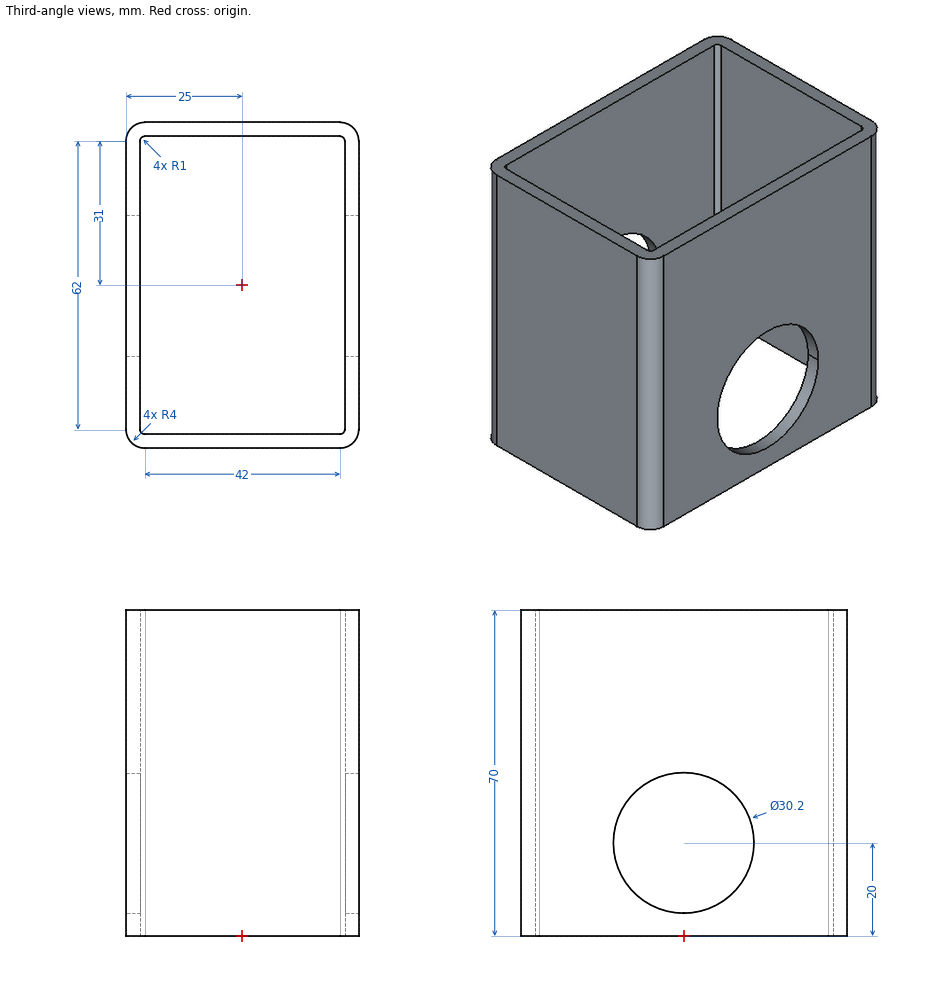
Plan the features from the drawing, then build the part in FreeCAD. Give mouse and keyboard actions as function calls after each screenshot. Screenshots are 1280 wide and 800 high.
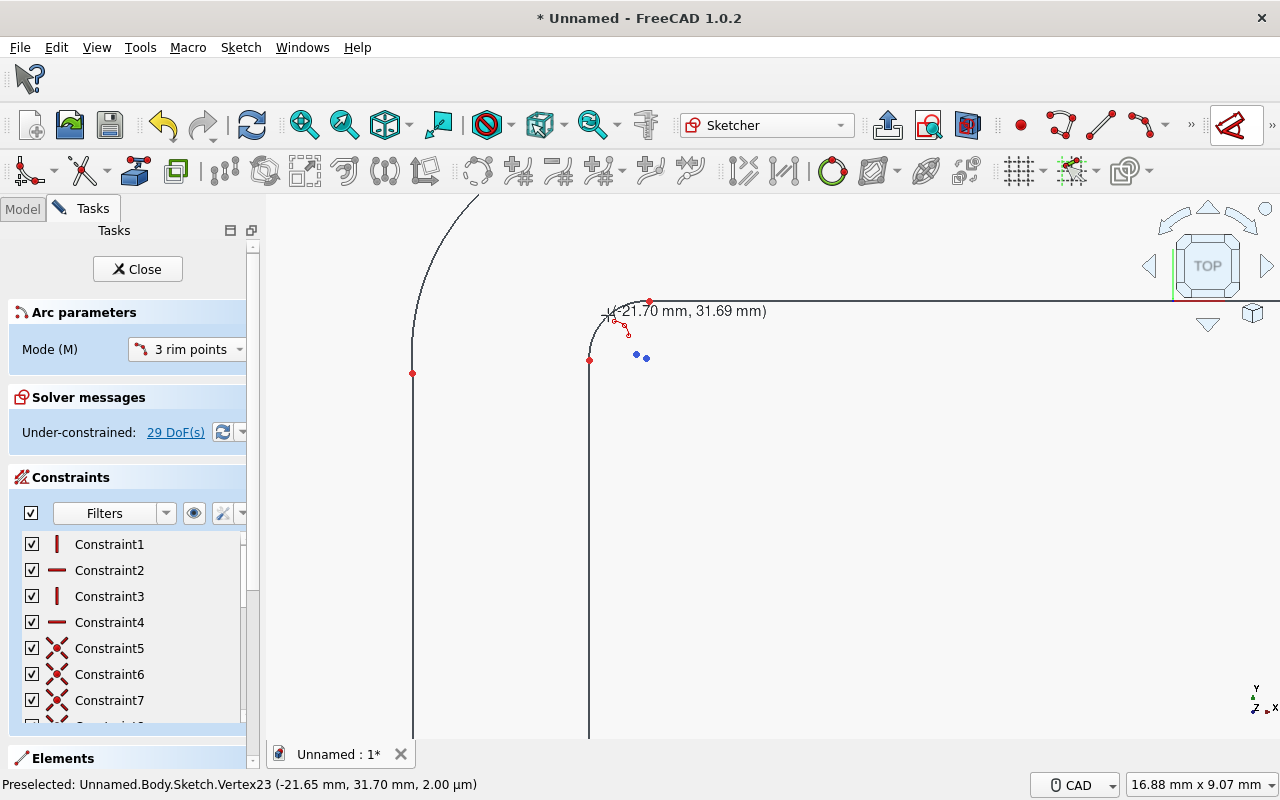
scroll(608, 326, down, 13)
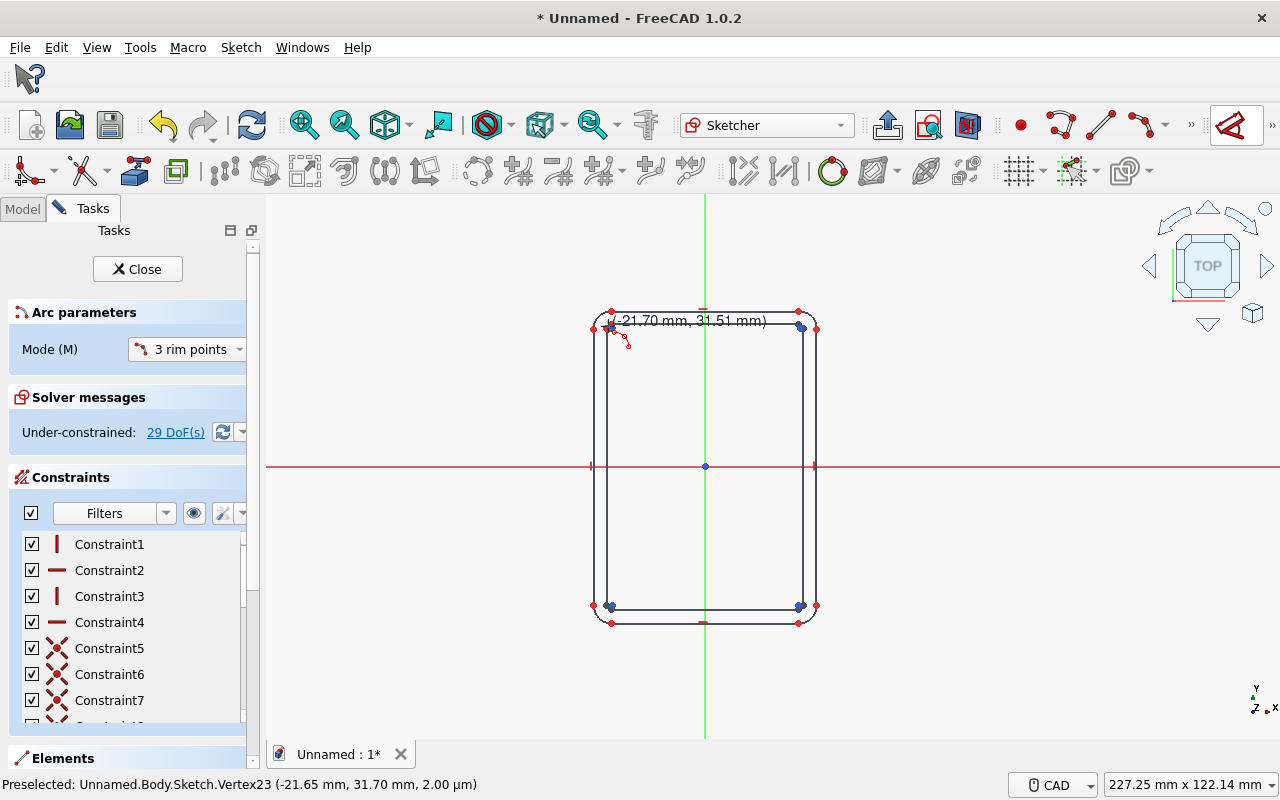
scroll(799, 324, up, 7)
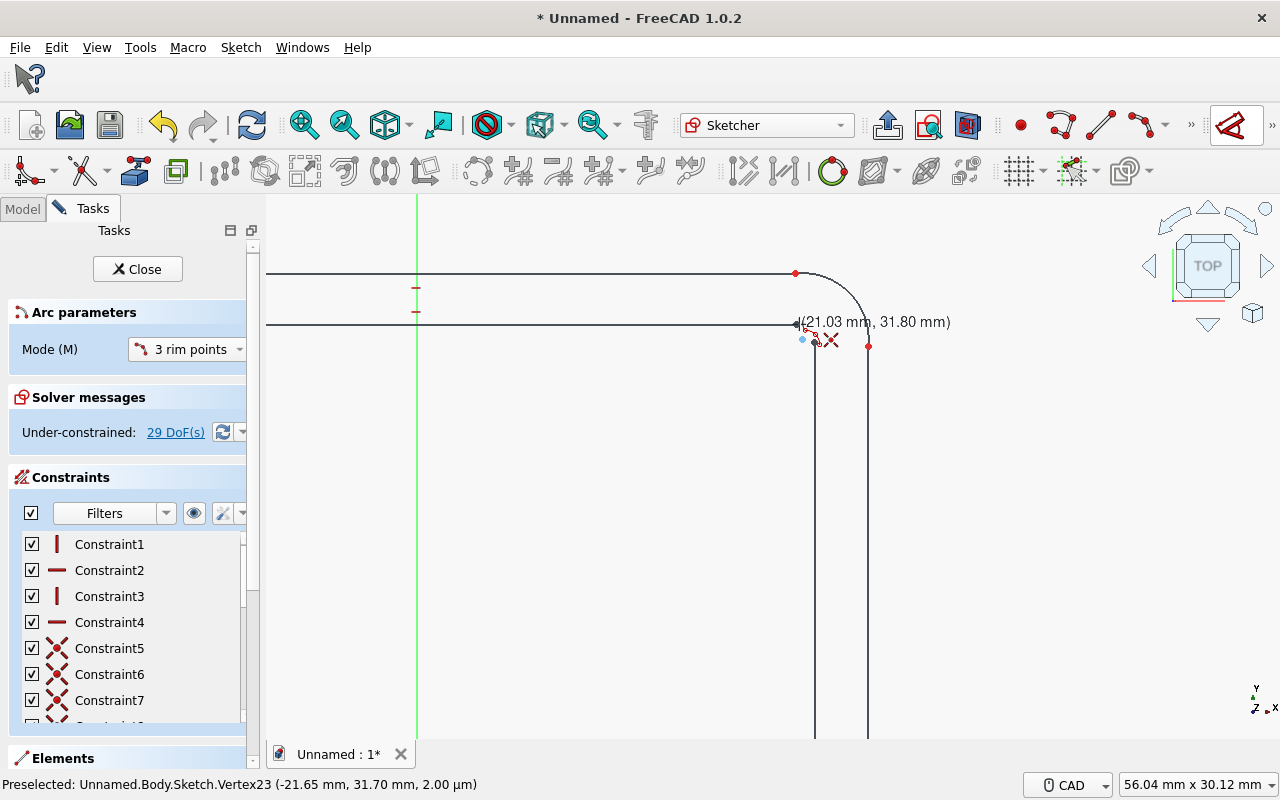
click(797, 325)
click(815, 343)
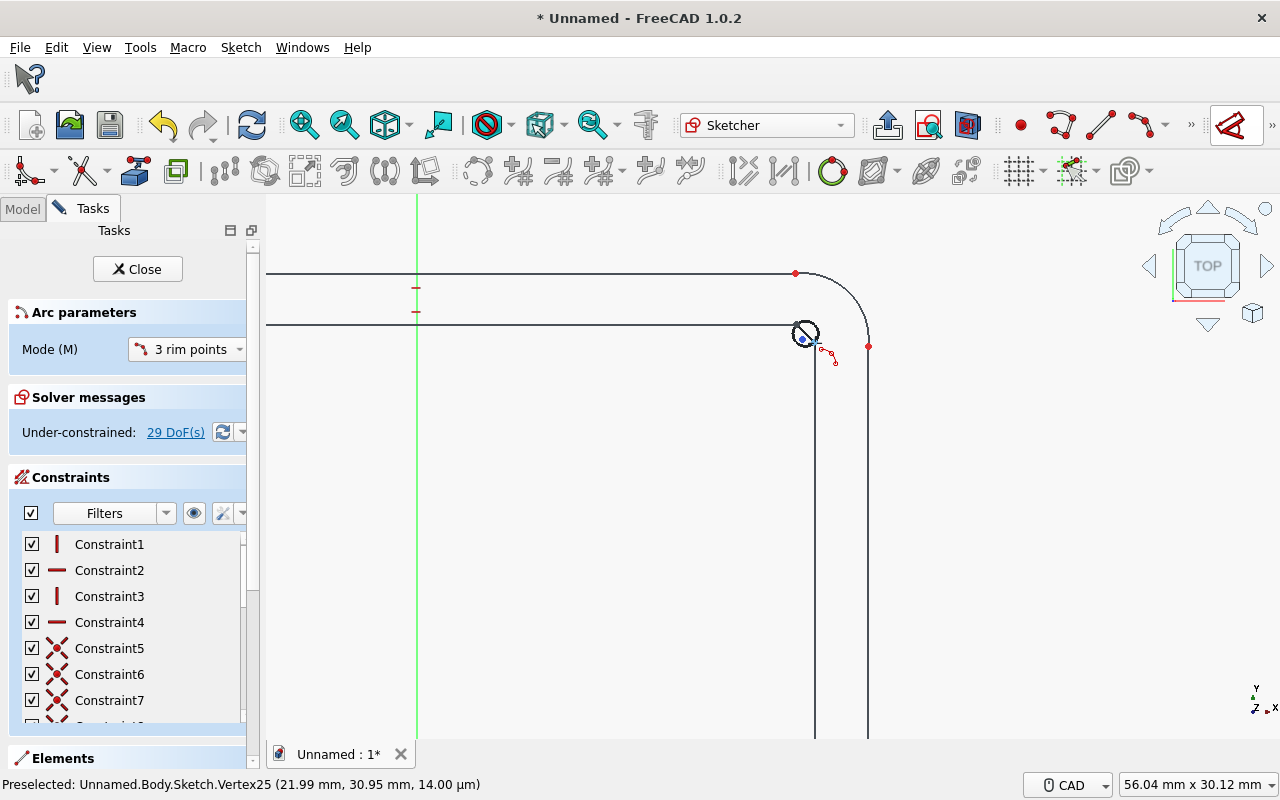
scroll(810, 329, up, 6)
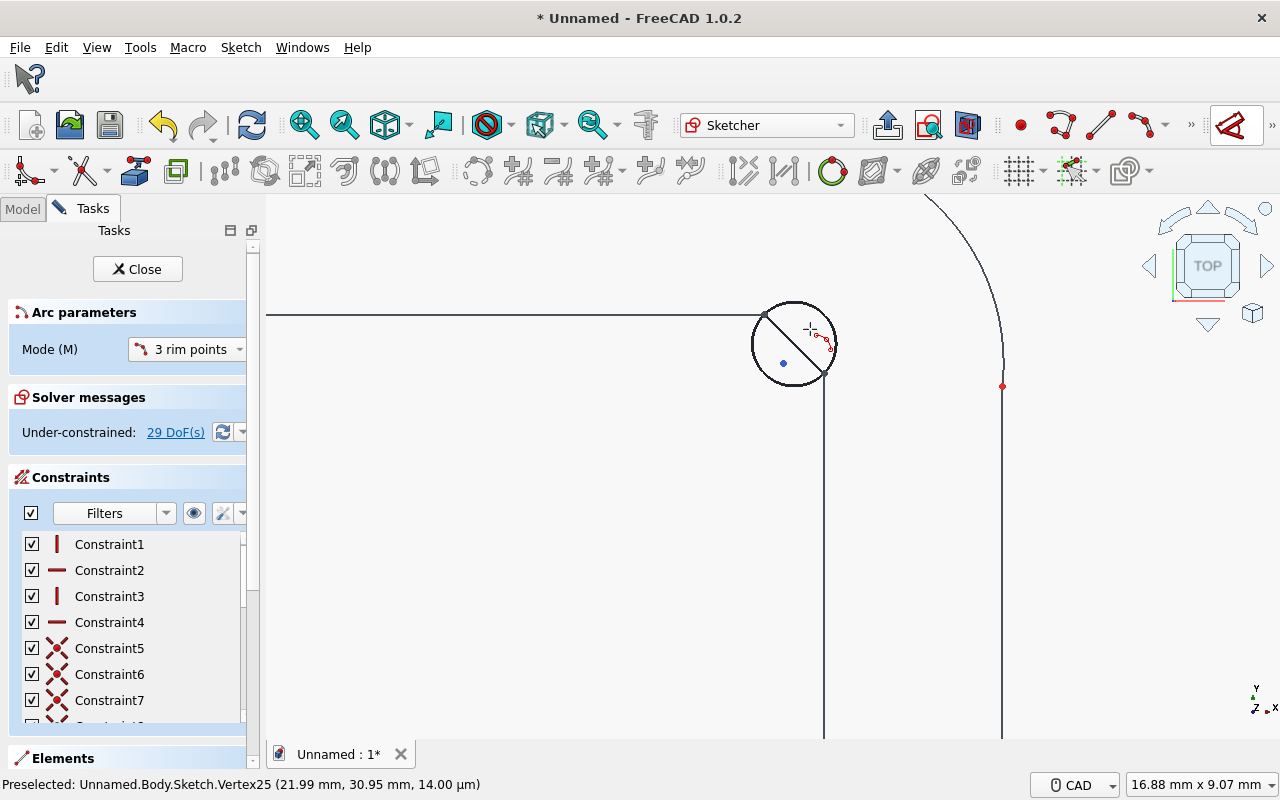
click(807, 328)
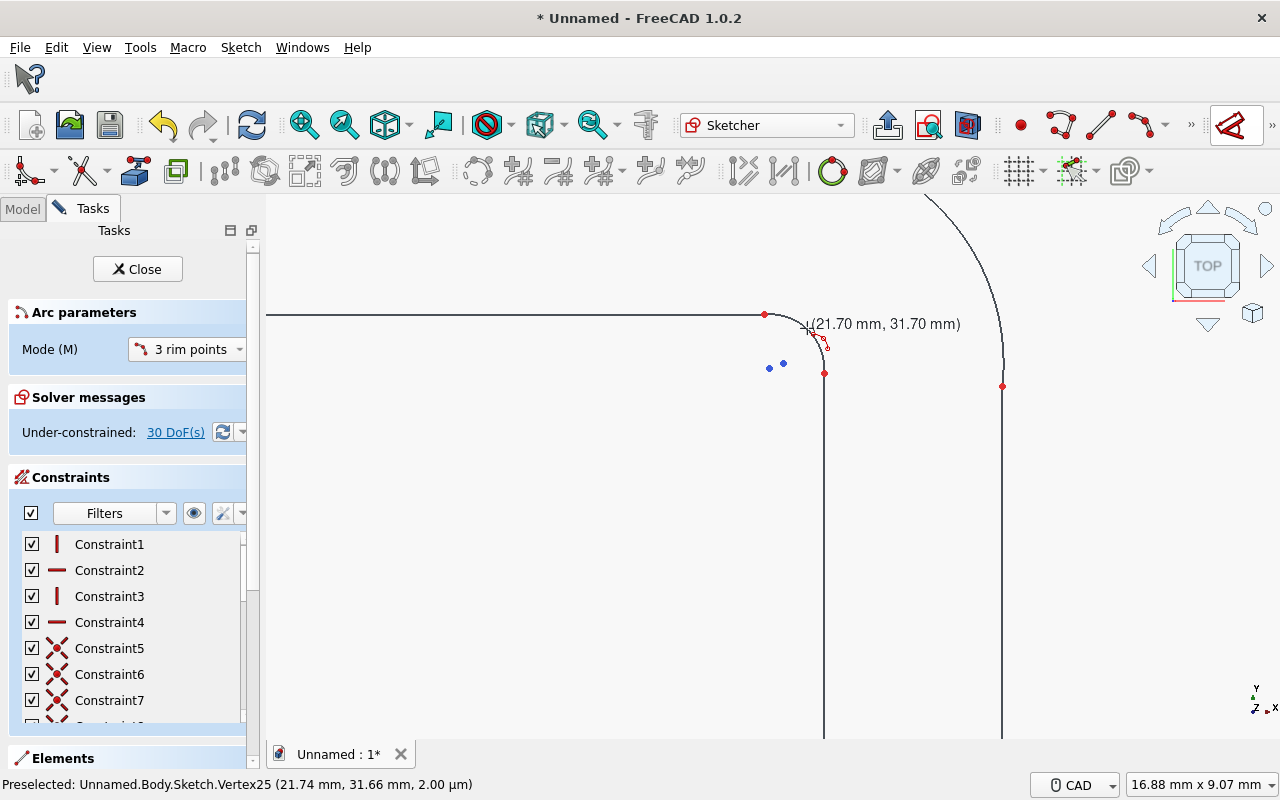
scroll(801, 325, down, 13)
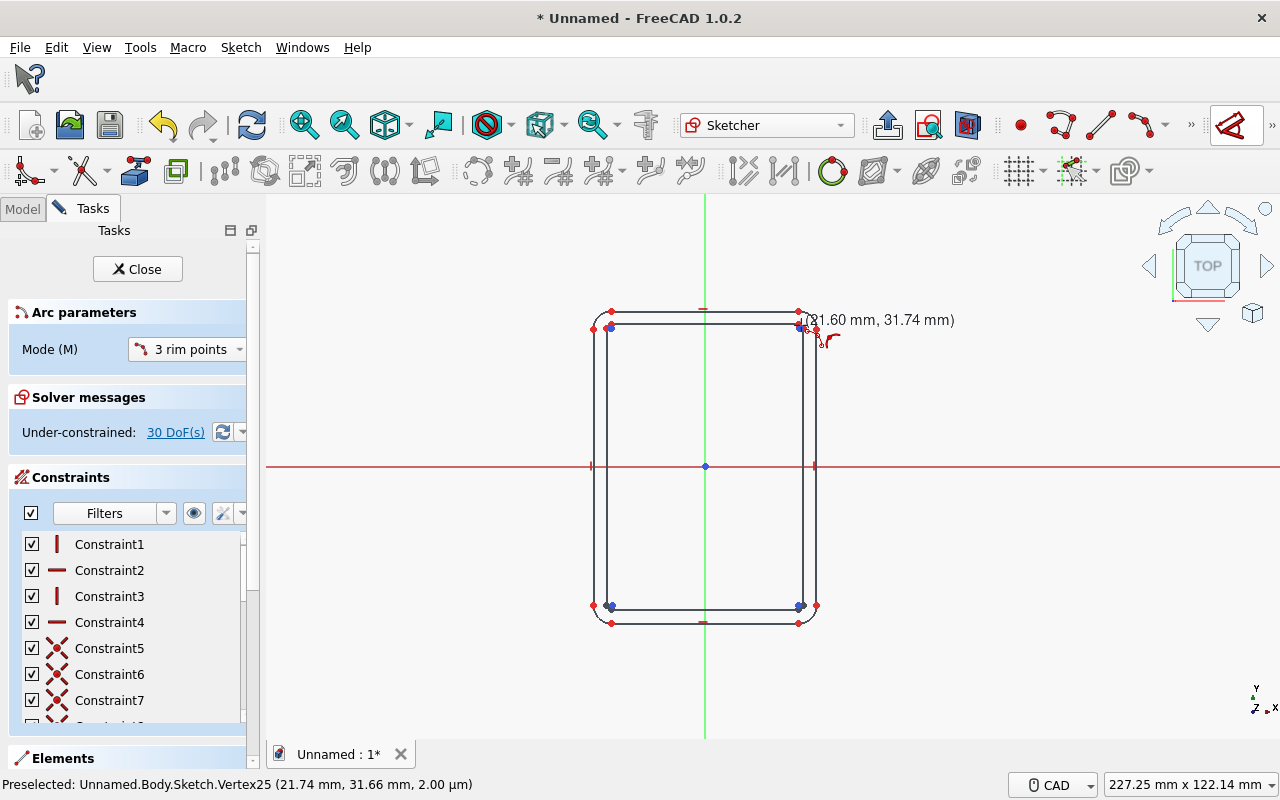
scroll(803, 605, up, 7)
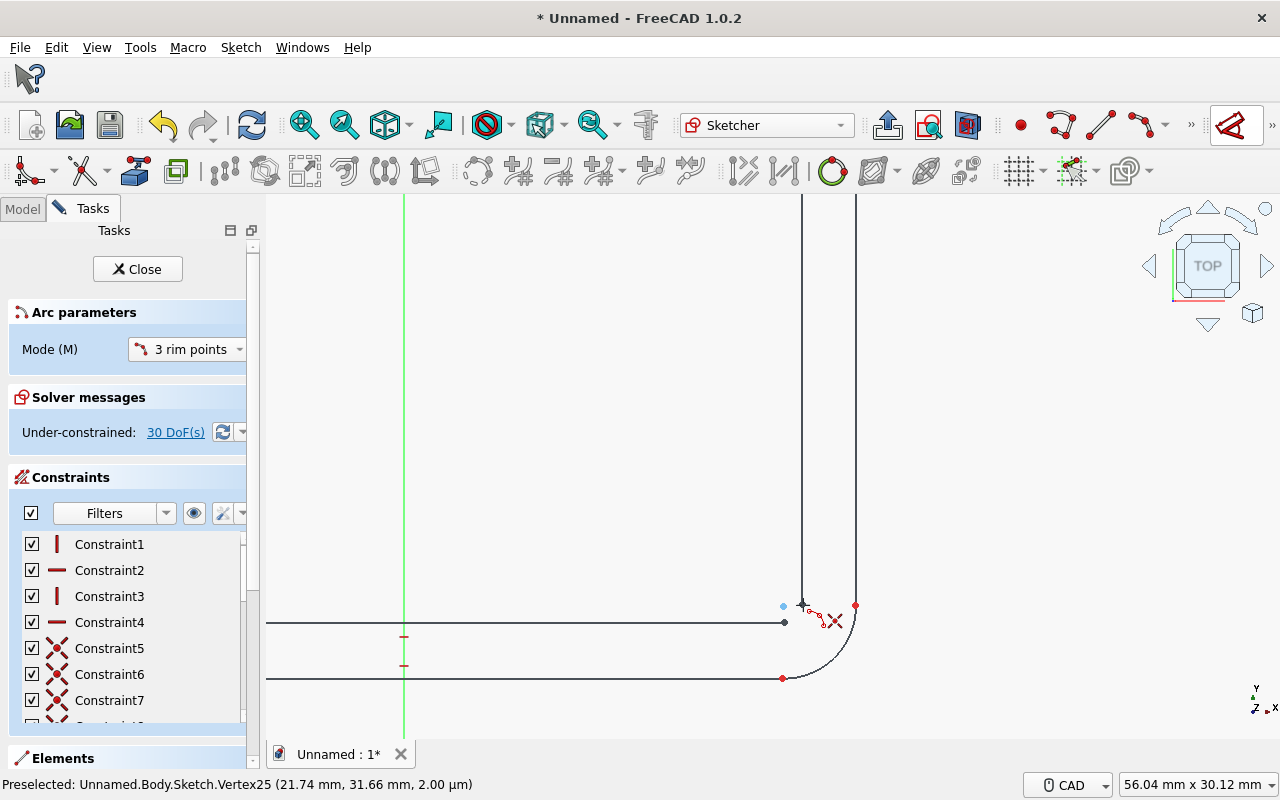
click(802, 605)
click(784, 623)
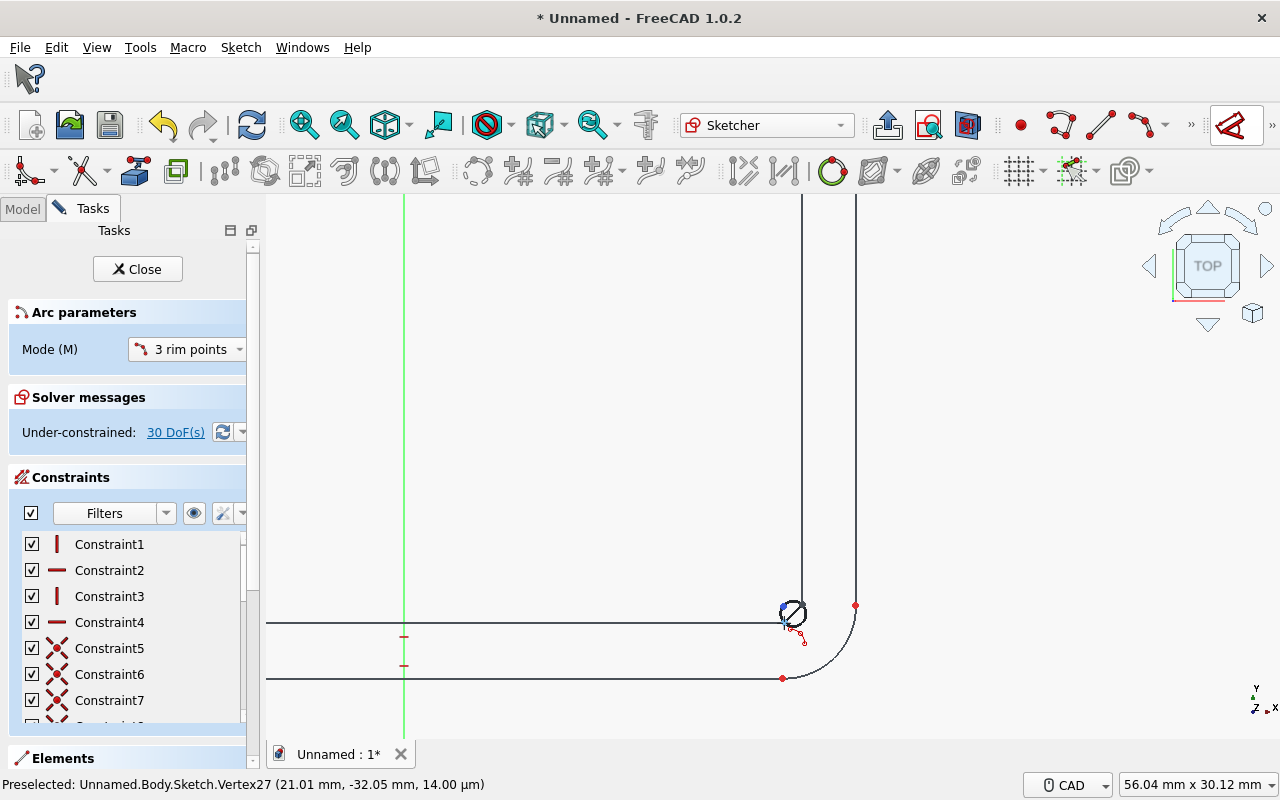
scroll(797, 617, up, 6)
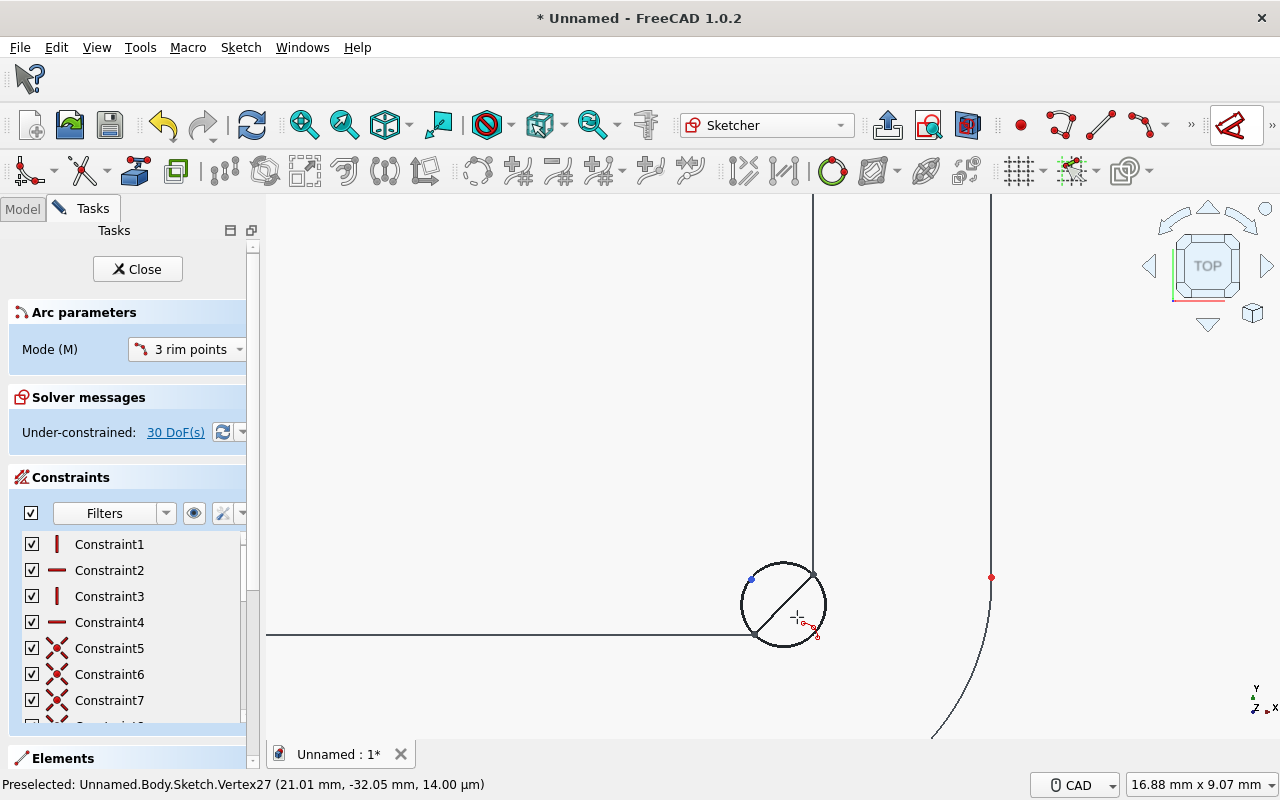
click(796, 614)